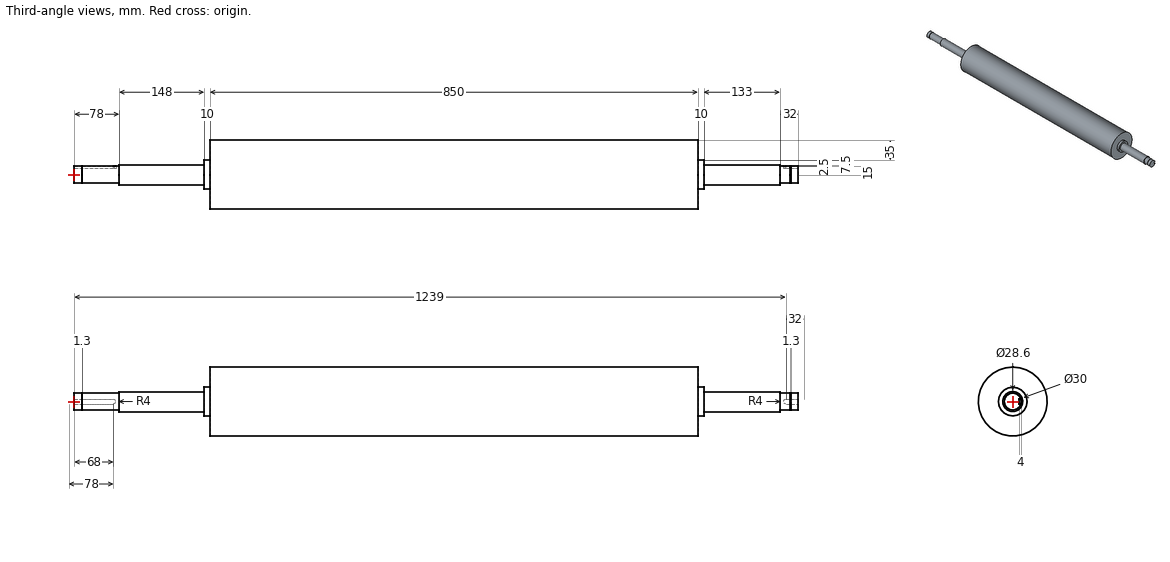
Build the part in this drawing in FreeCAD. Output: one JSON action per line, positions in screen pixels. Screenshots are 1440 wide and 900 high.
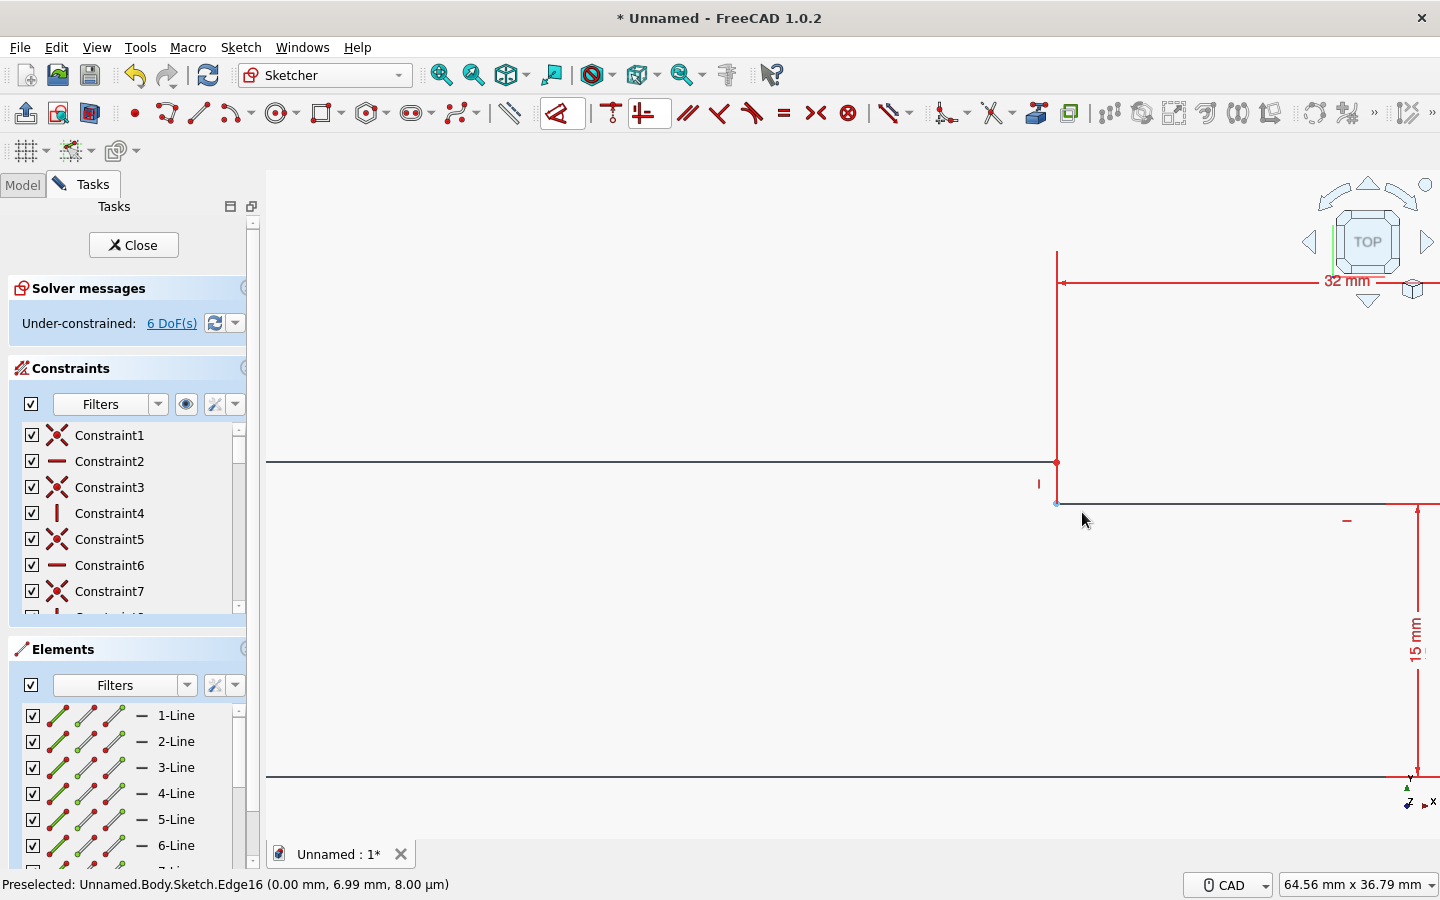
{"action": "left_click", "coordinate": [1057, 483]}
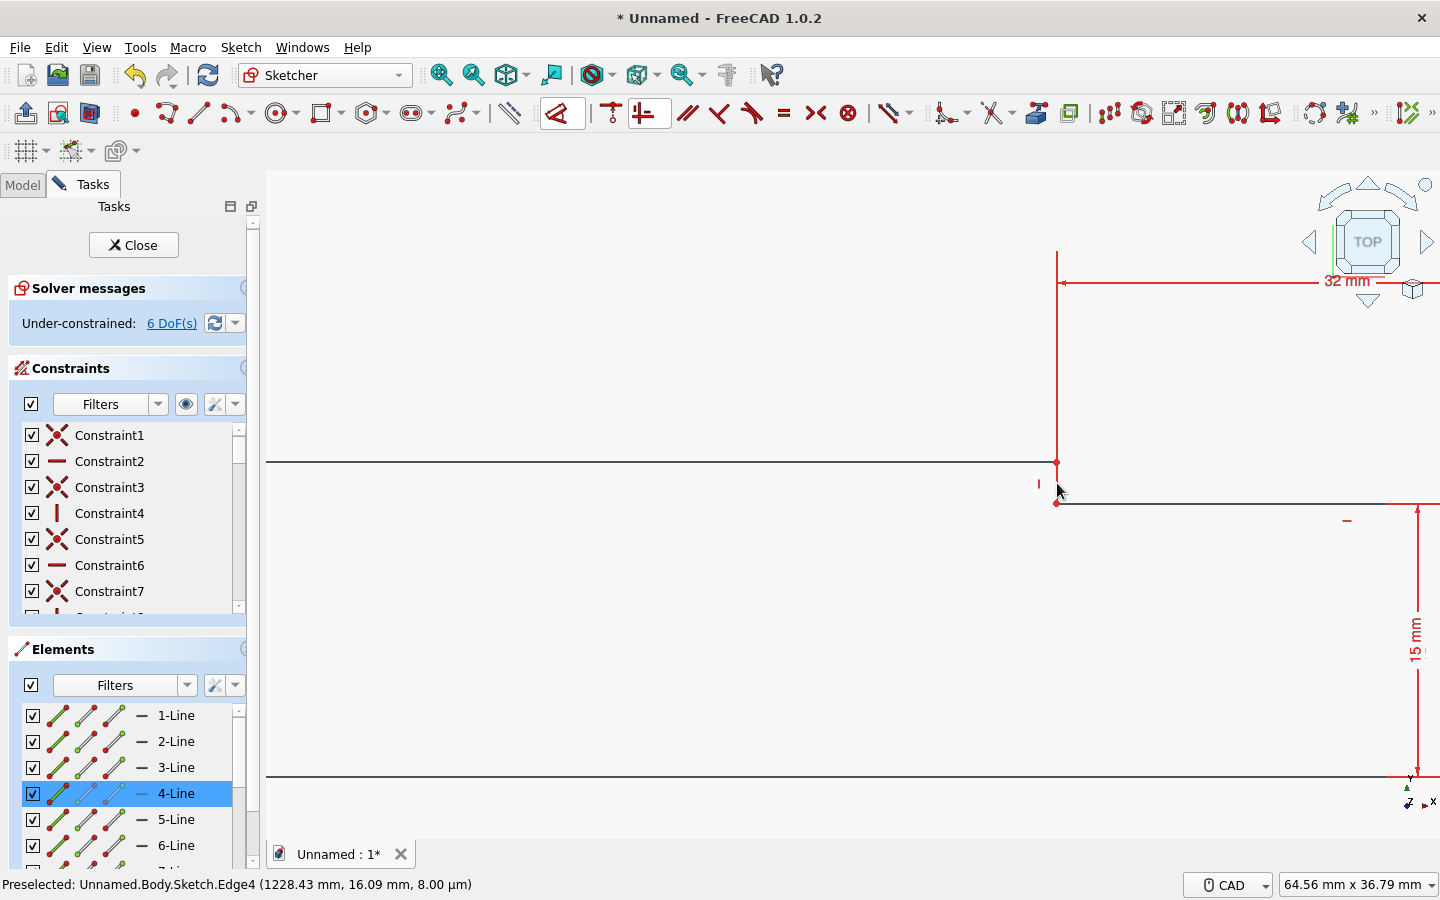
{"action": "key", "text": "i"}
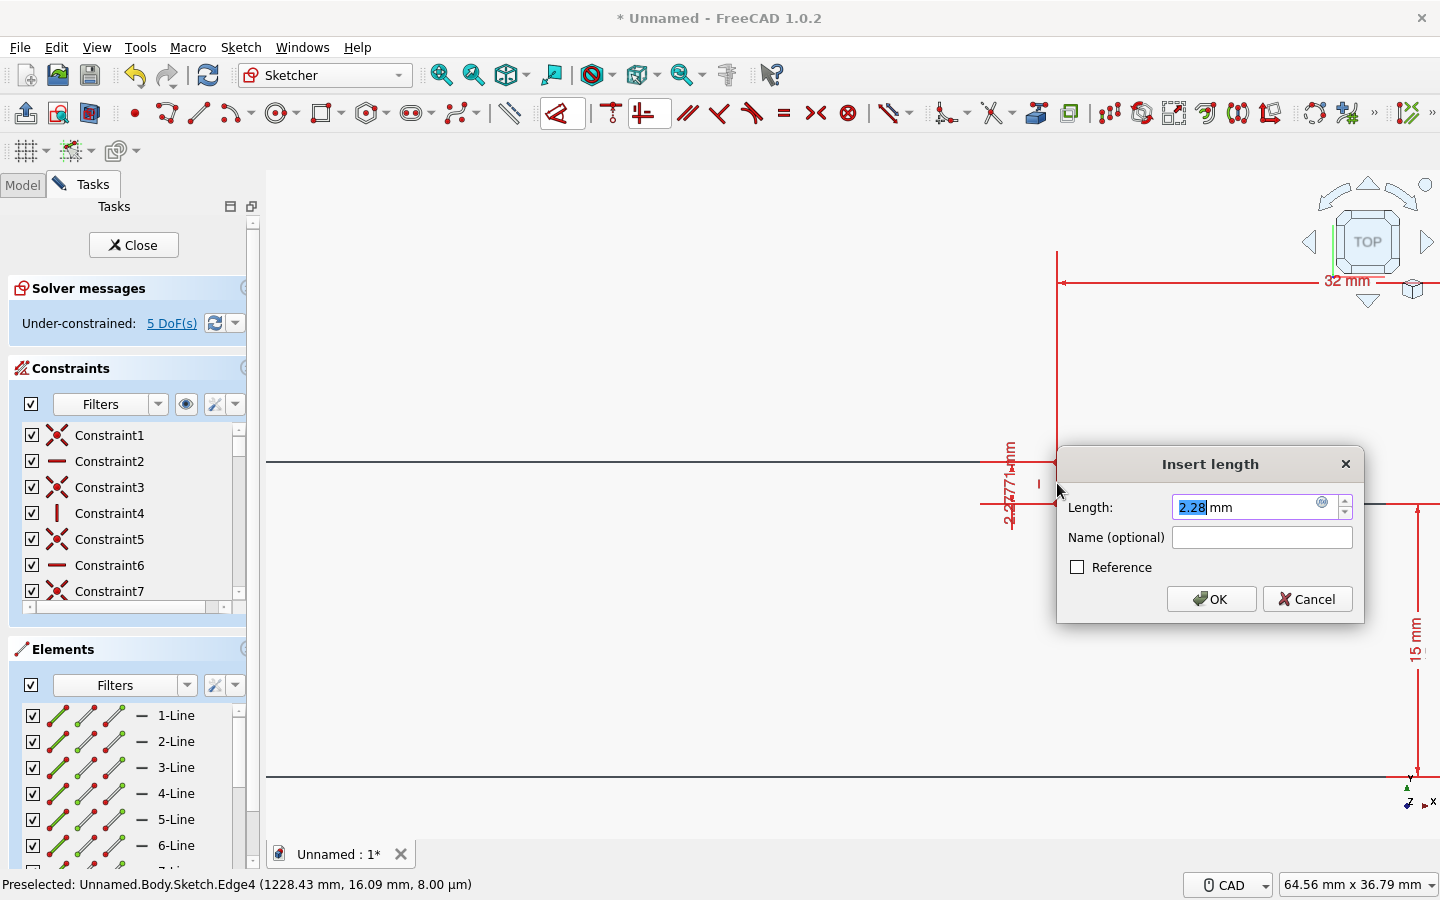
{"action": "type", "text": "2.5"}
{"action": "key", "text": "Return"}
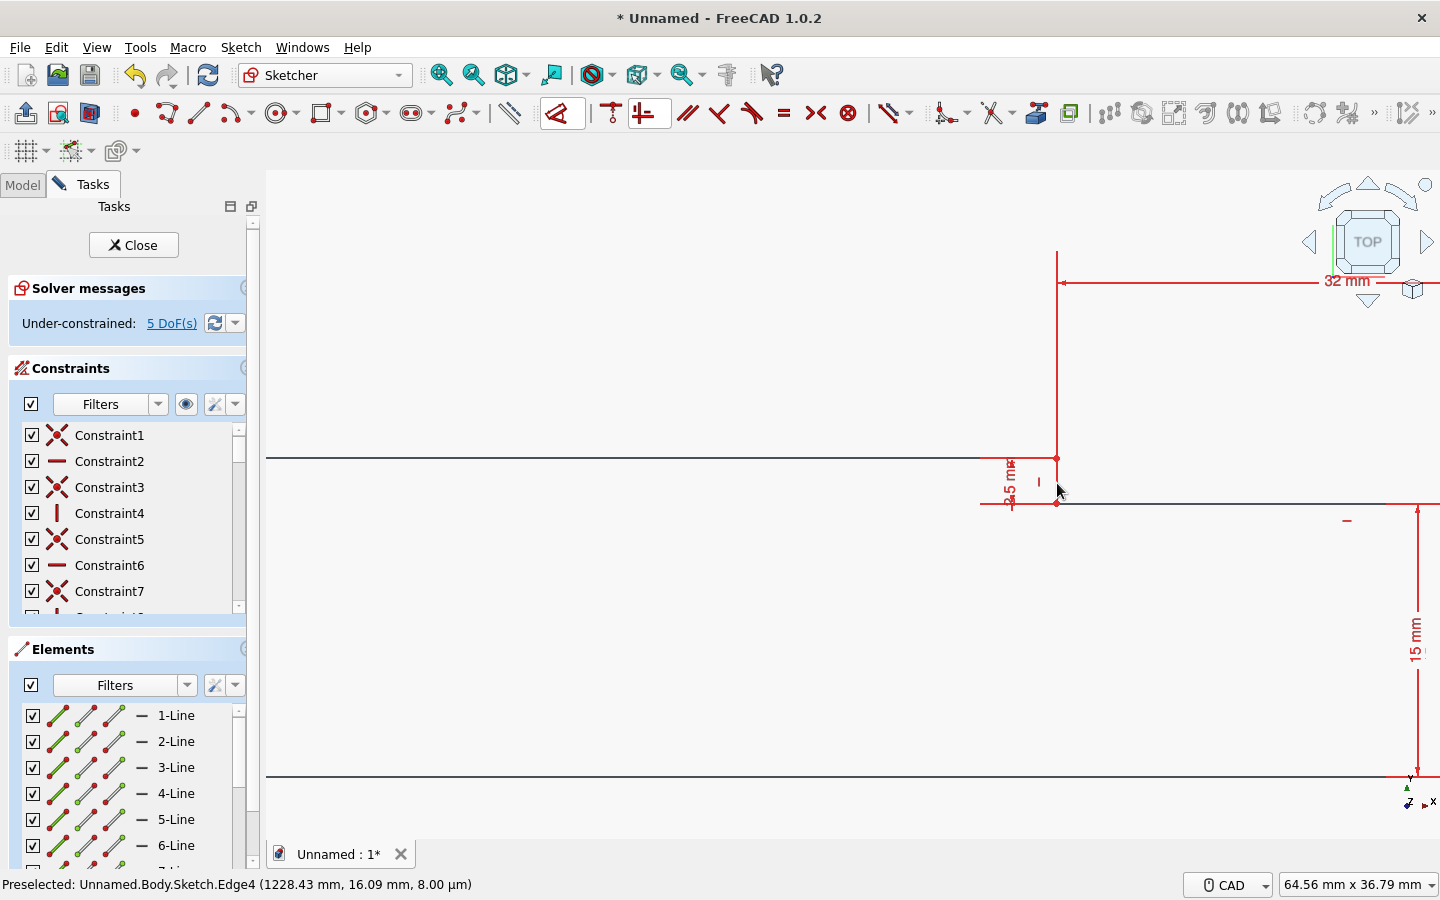
{"action": "scroll", "coordinate": [1151, 514], "scroll_direction": "down", "scroll_amount": 17}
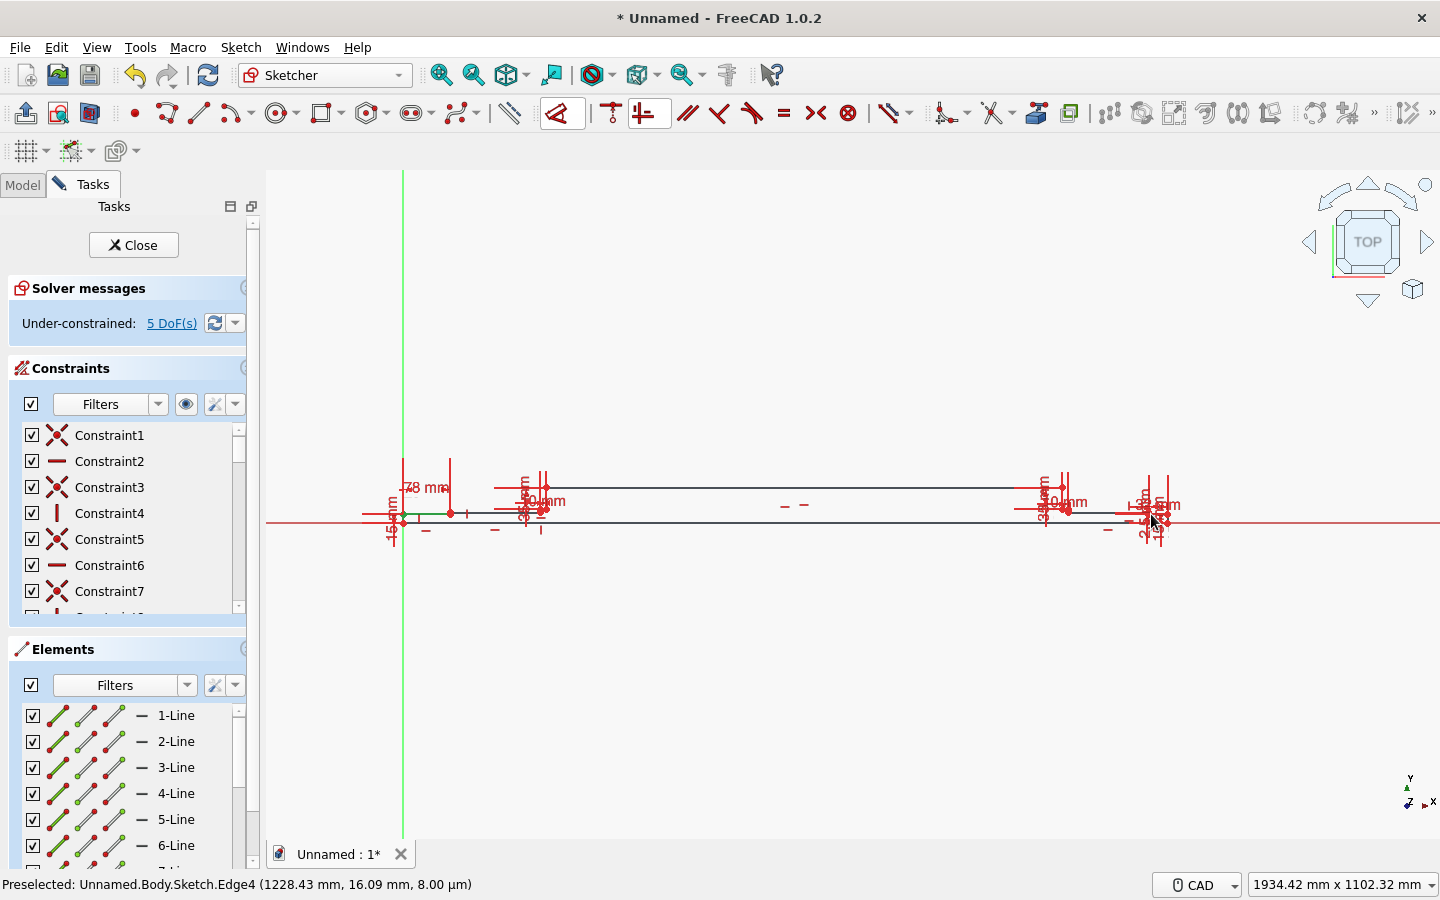
{"action": "scroll", "coordinate": [1124, 513], "scroll_direction": "up", "scroll_amount": 2}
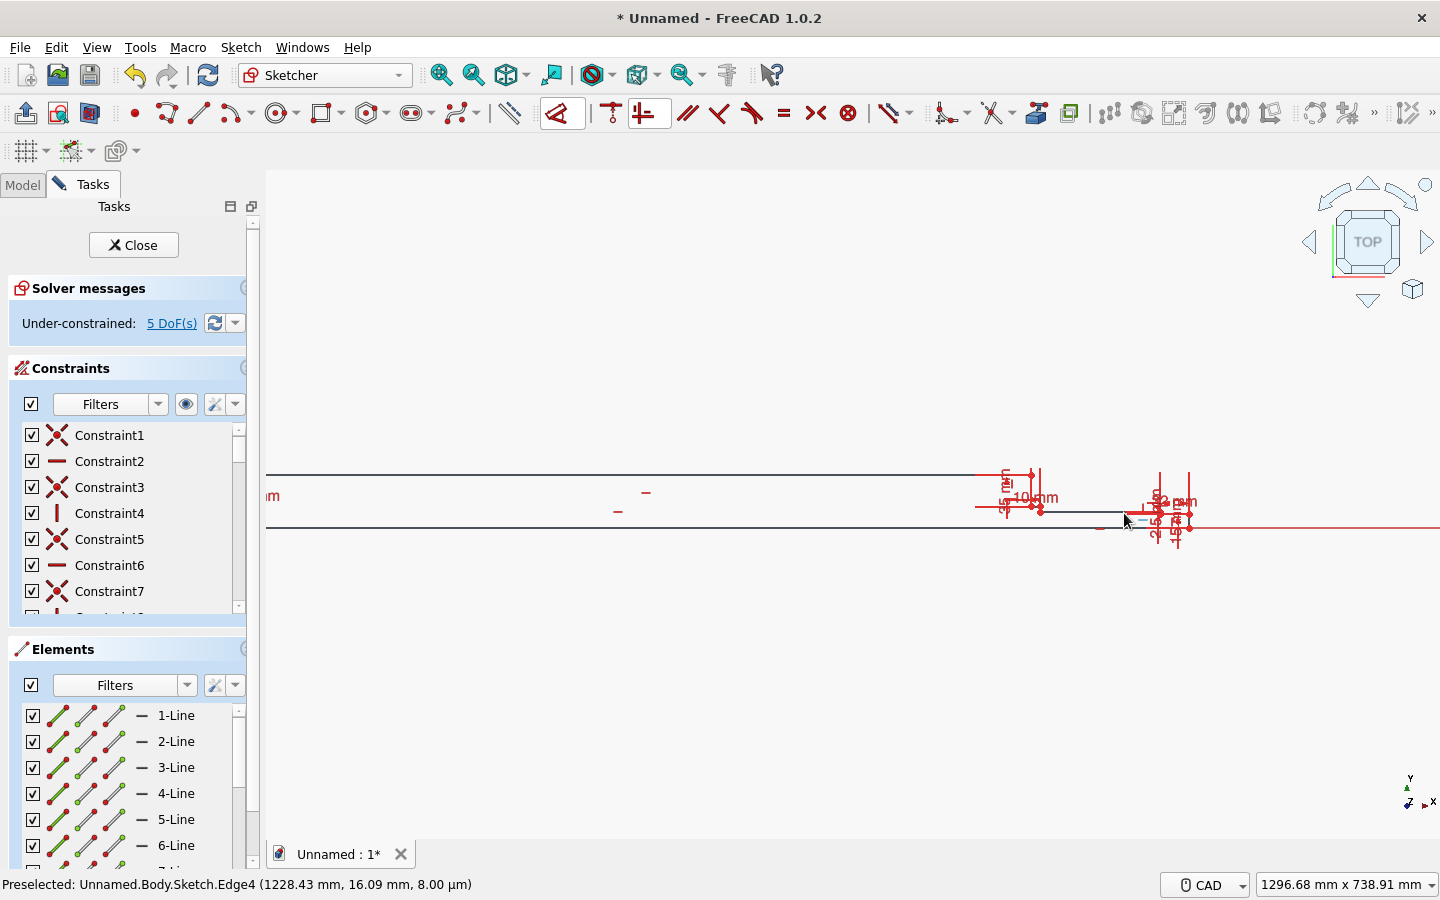
{"action": "left_click", "coordinate": [1124, 512]}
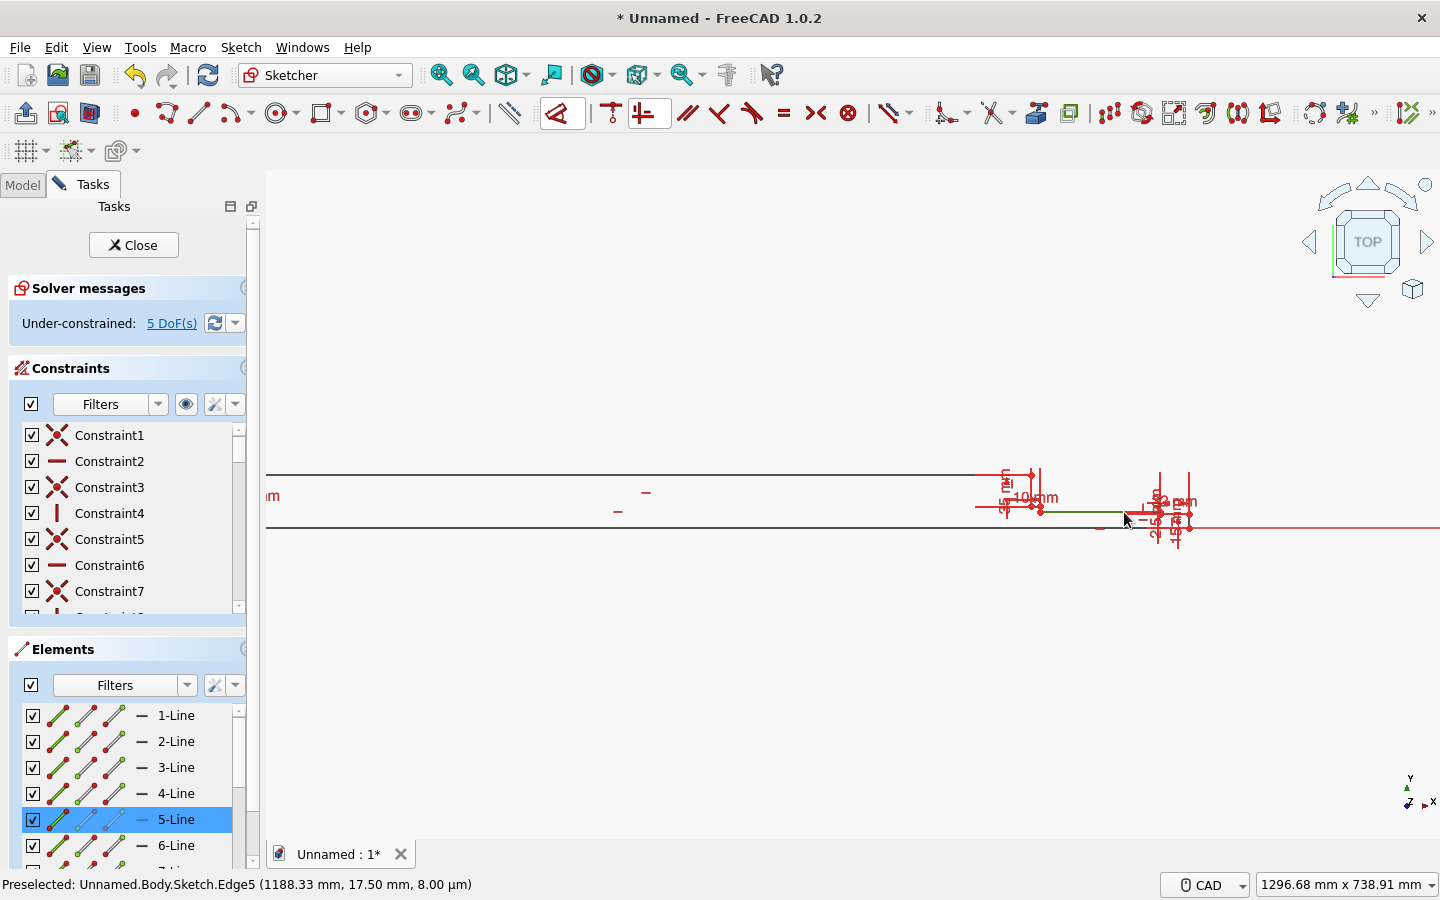
{"action": "left_click", "coordinate": [580, 114]}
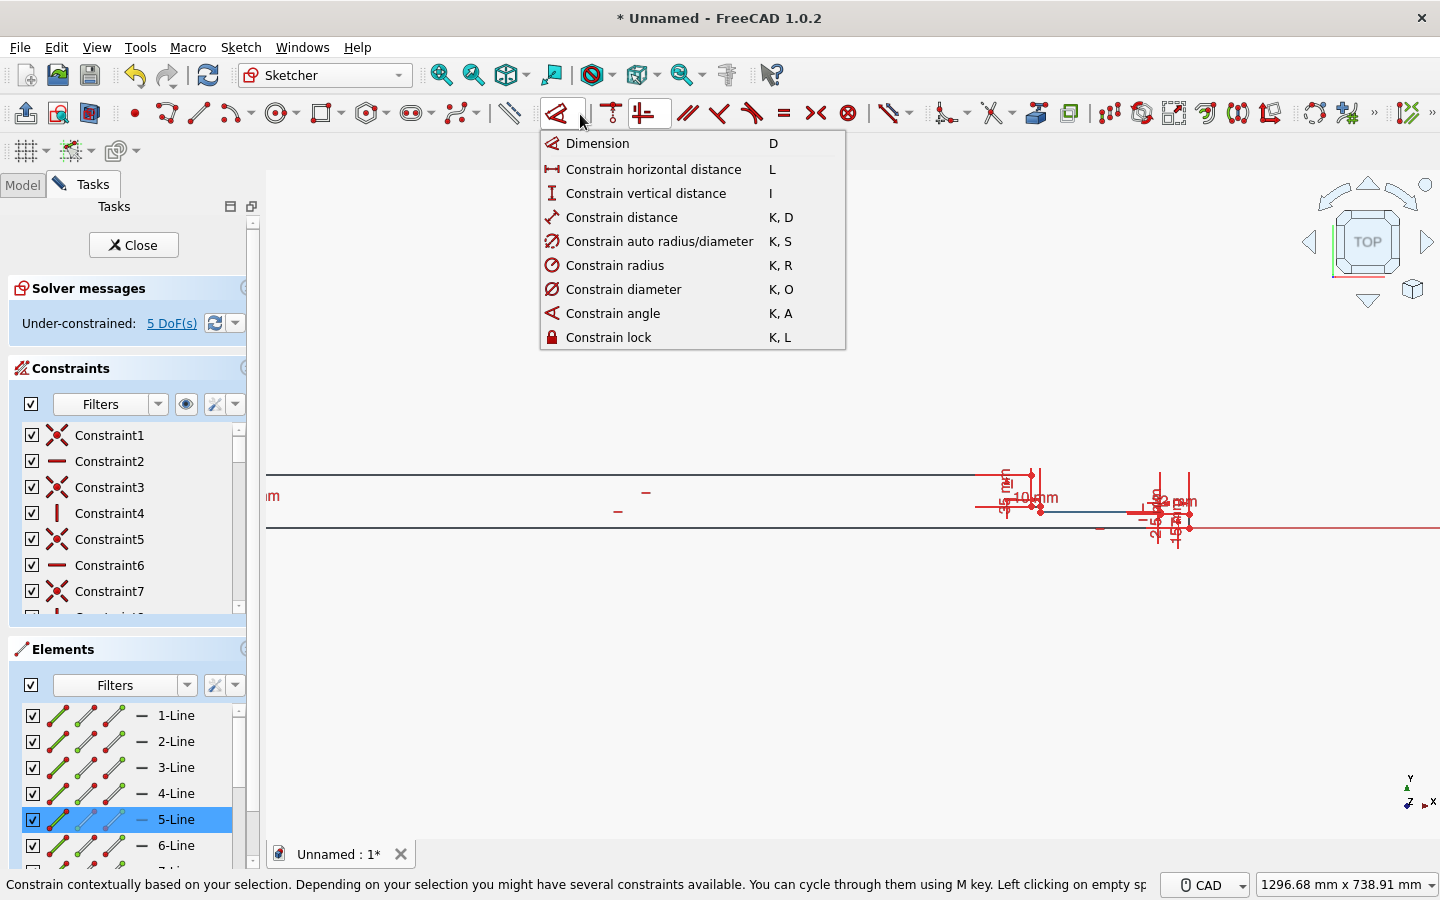
{"action": "left_click", "coordinate": [693, 169]}